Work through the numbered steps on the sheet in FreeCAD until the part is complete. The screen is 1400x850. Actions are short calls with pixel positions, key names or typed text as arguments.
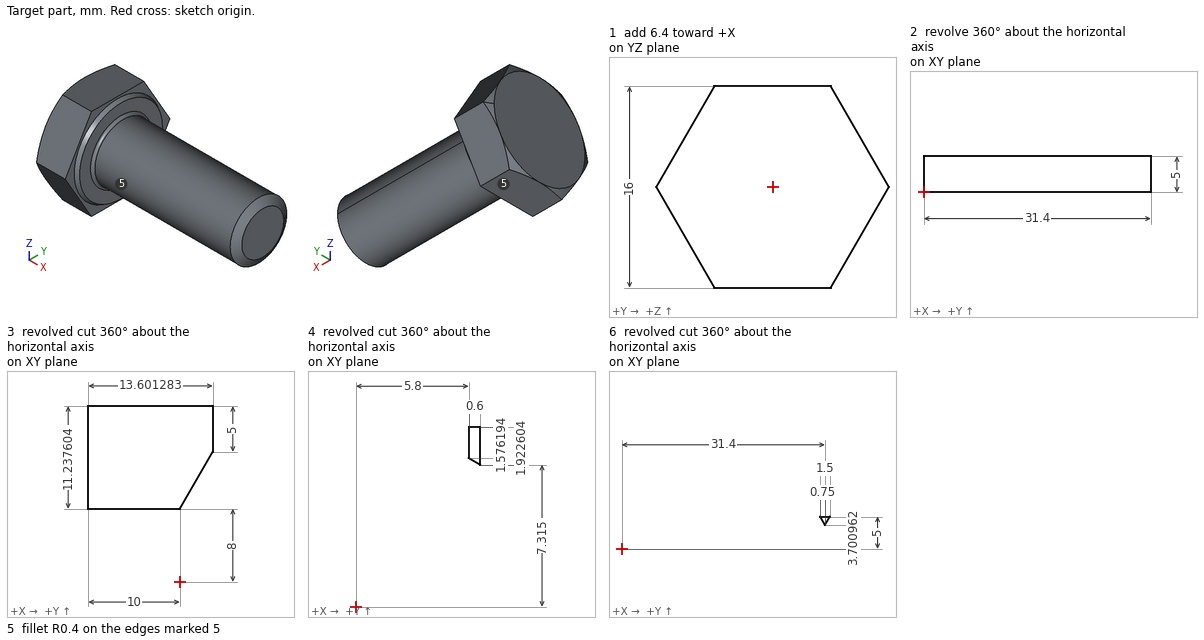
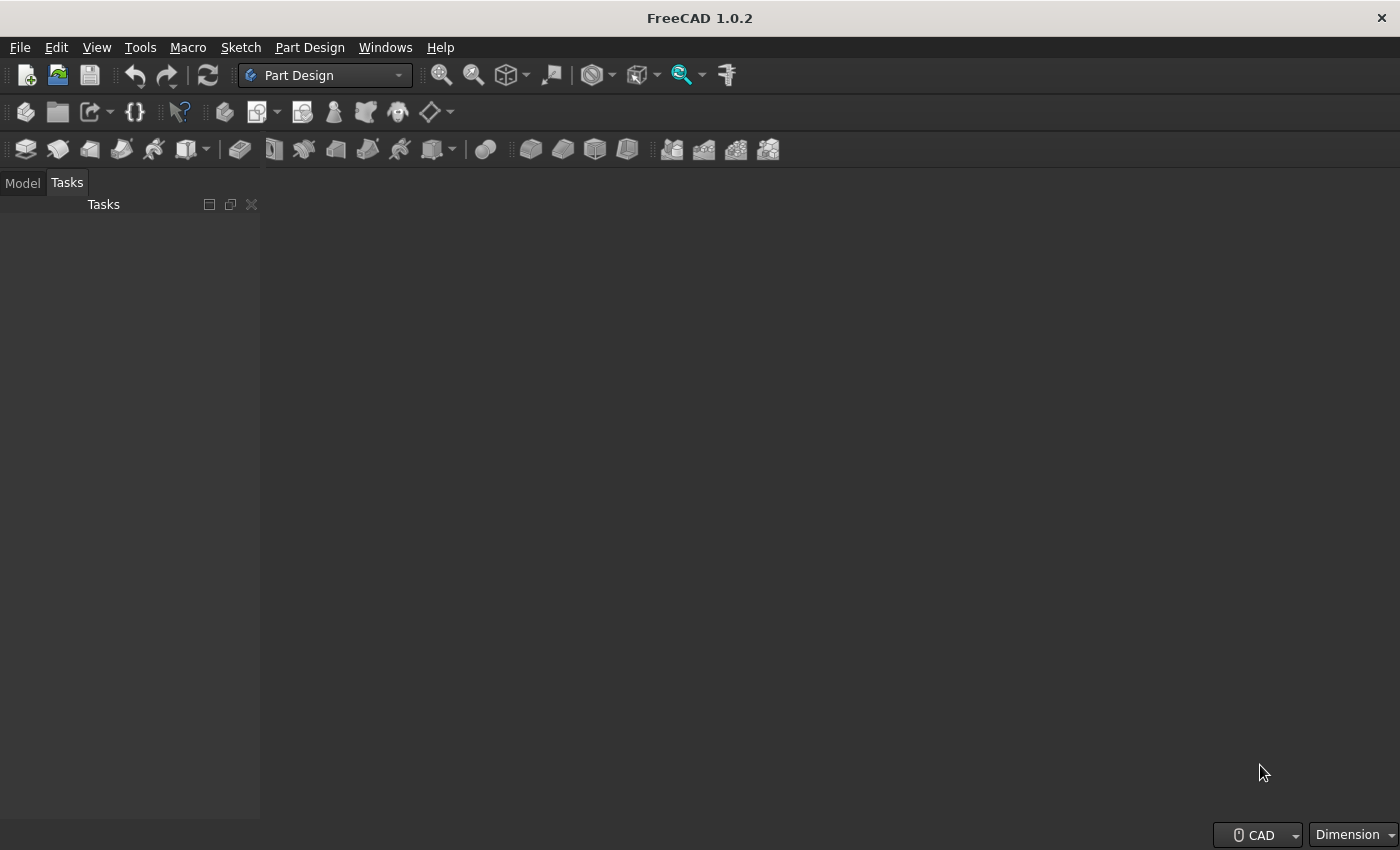
click(26, 76)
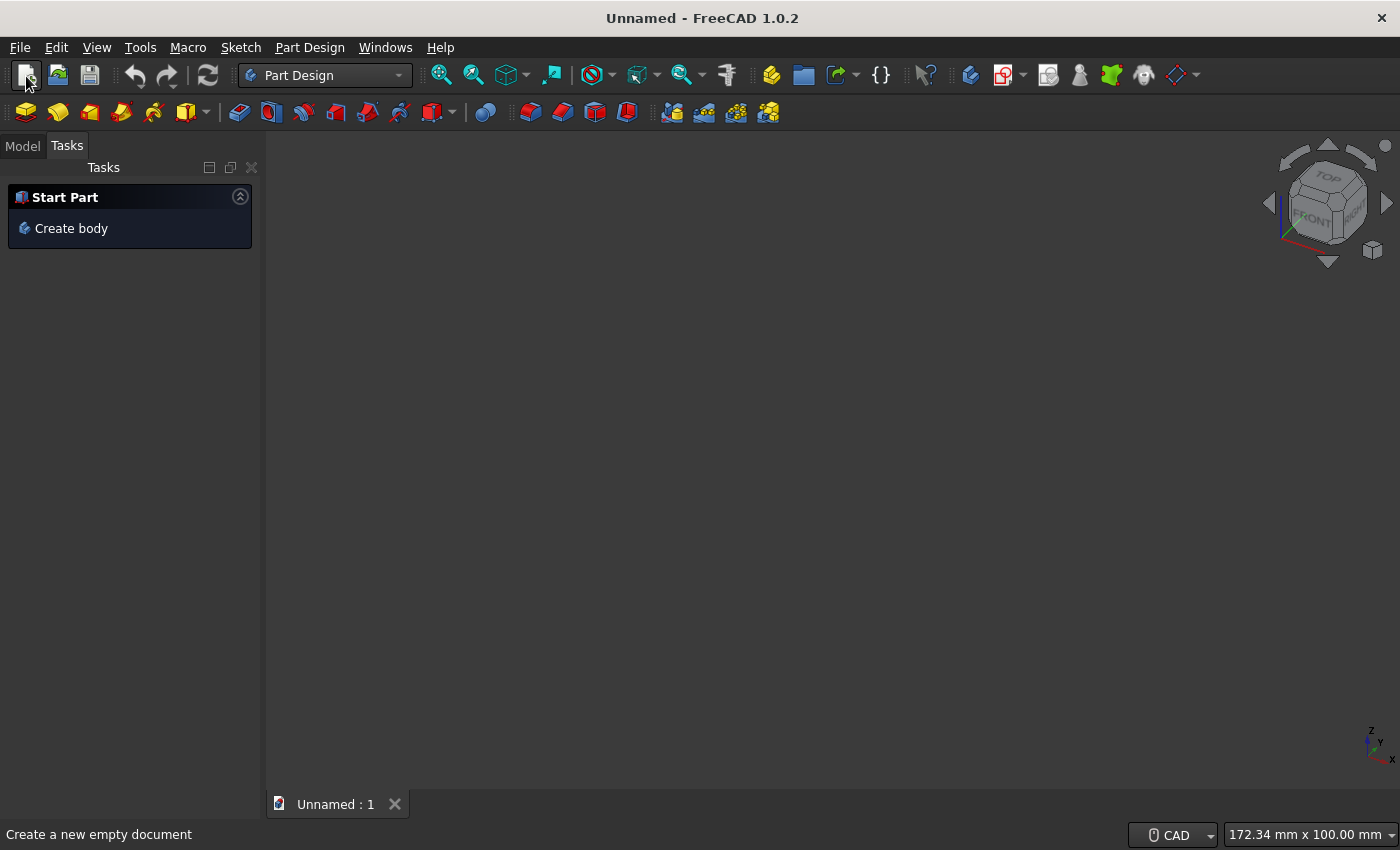
click(1004, 76)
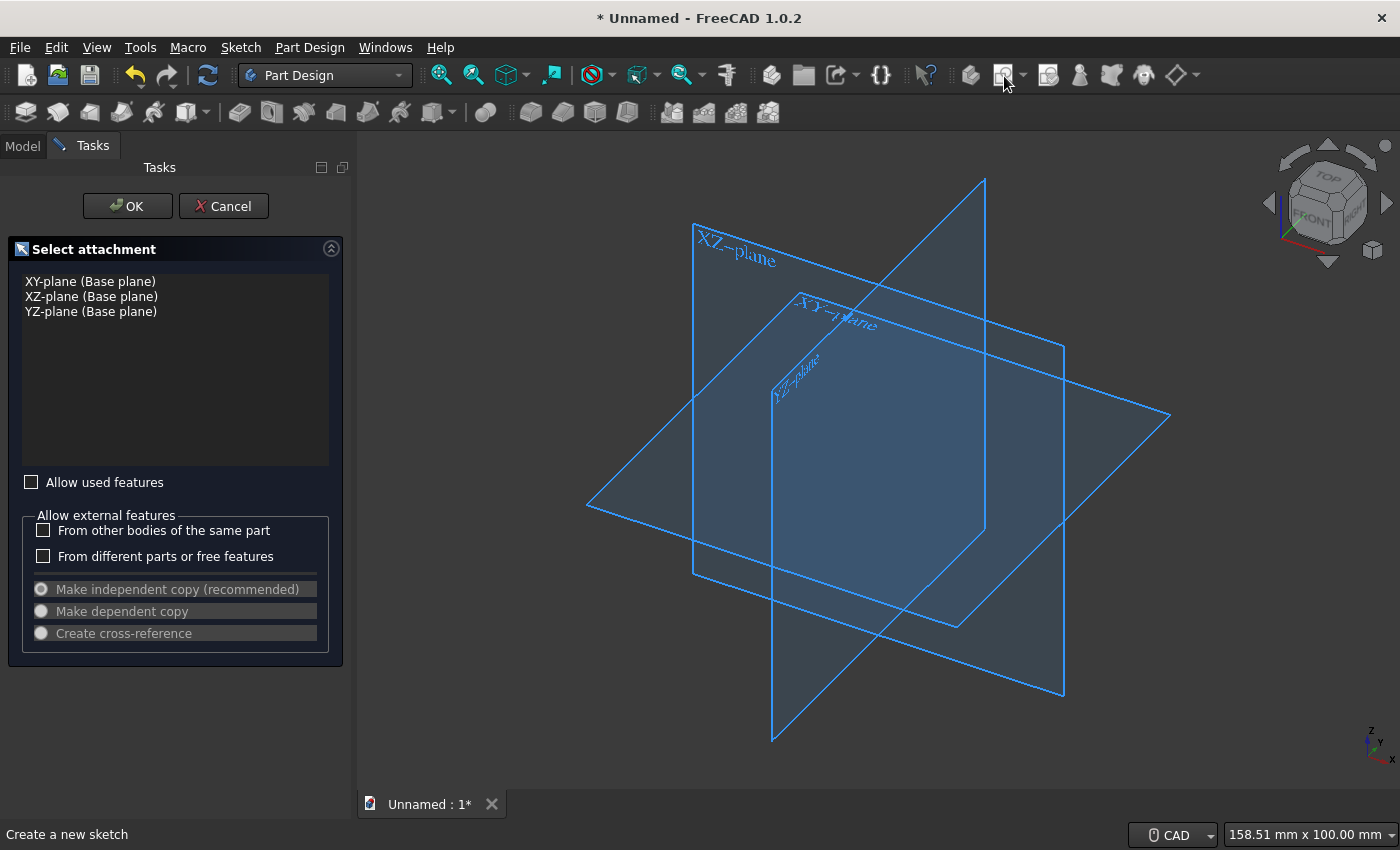
click(82, 312)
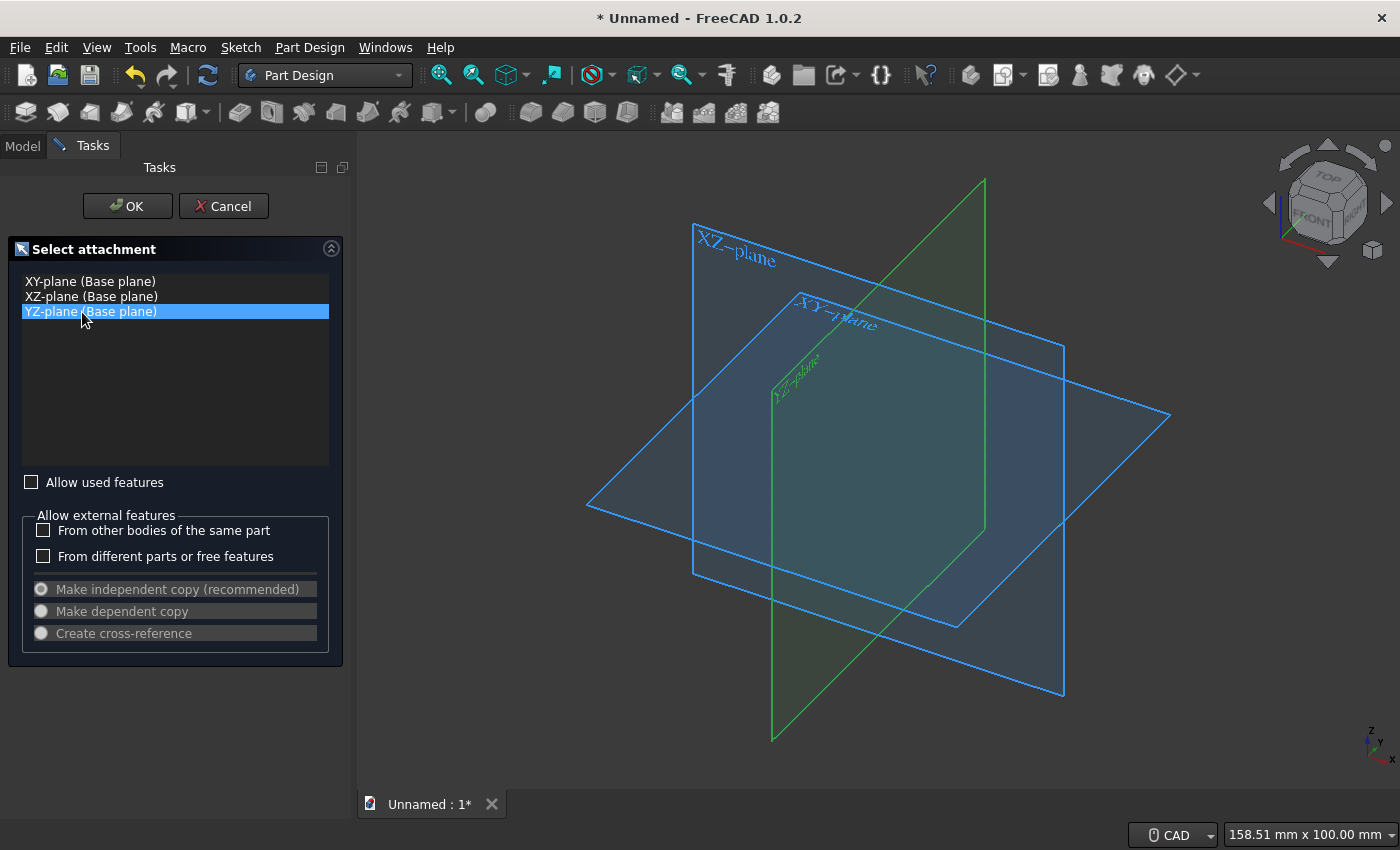
click(128, 206)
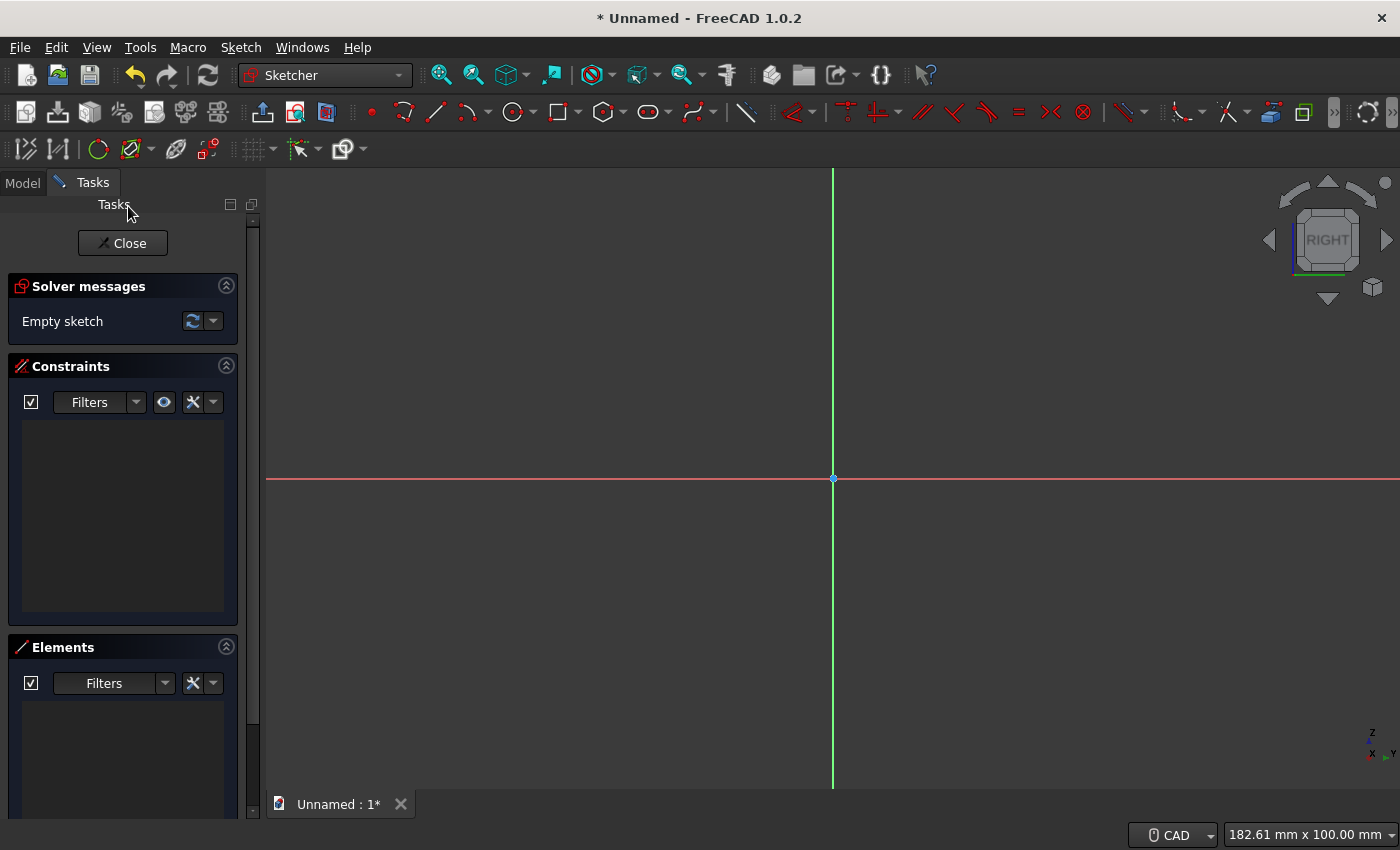
scroll(855, 479, up, 7)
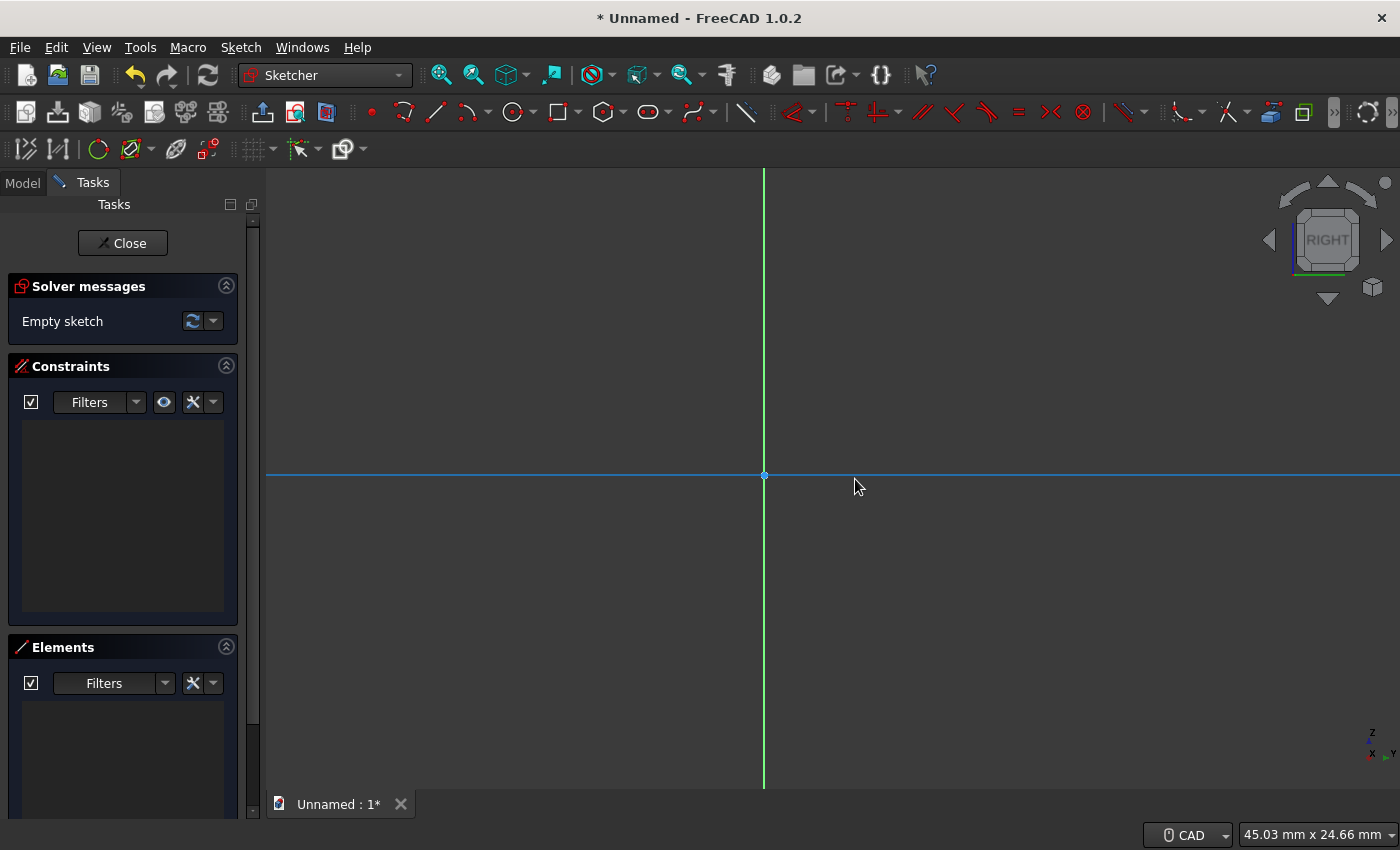
click(604, 112)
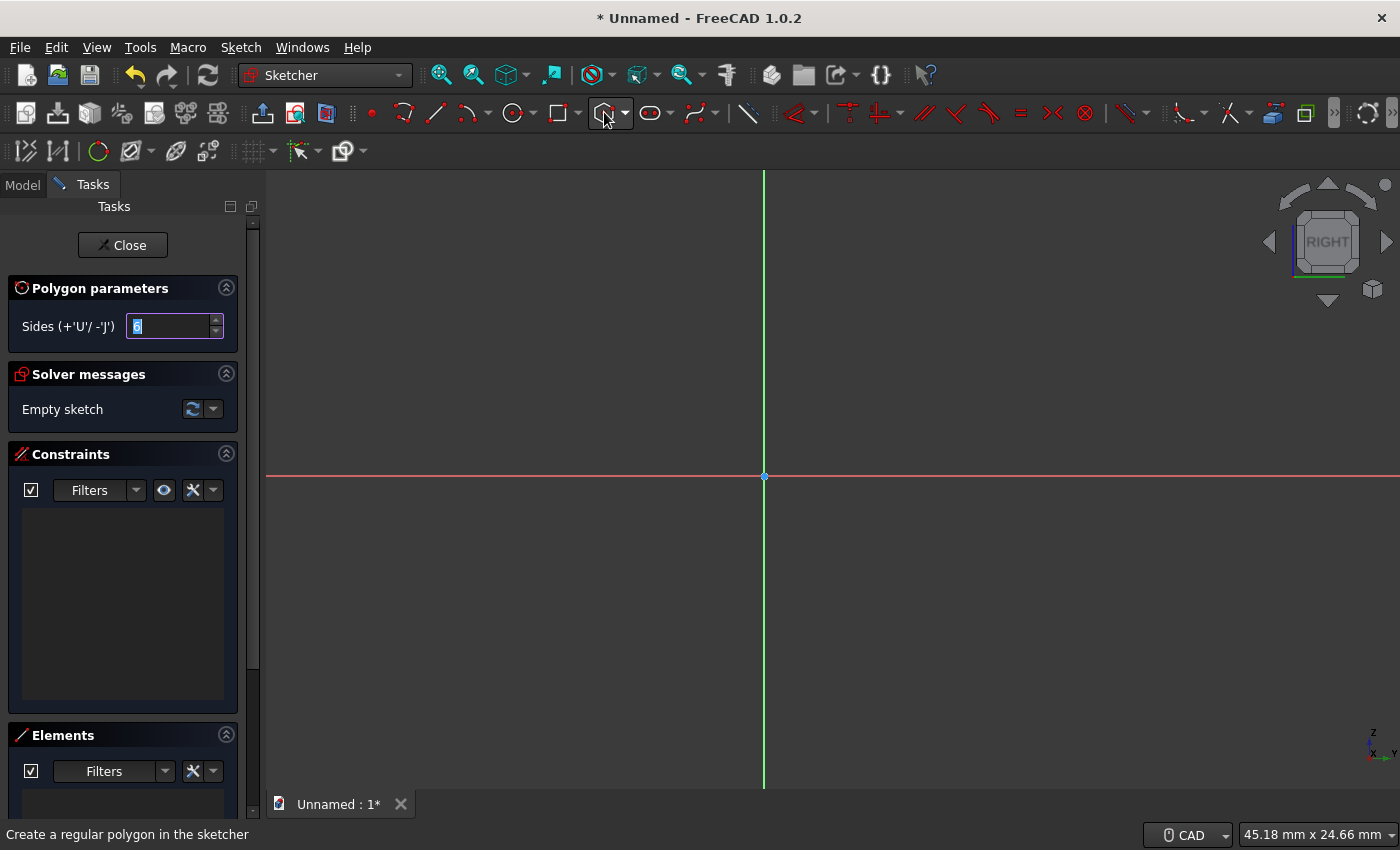
click(764, 476)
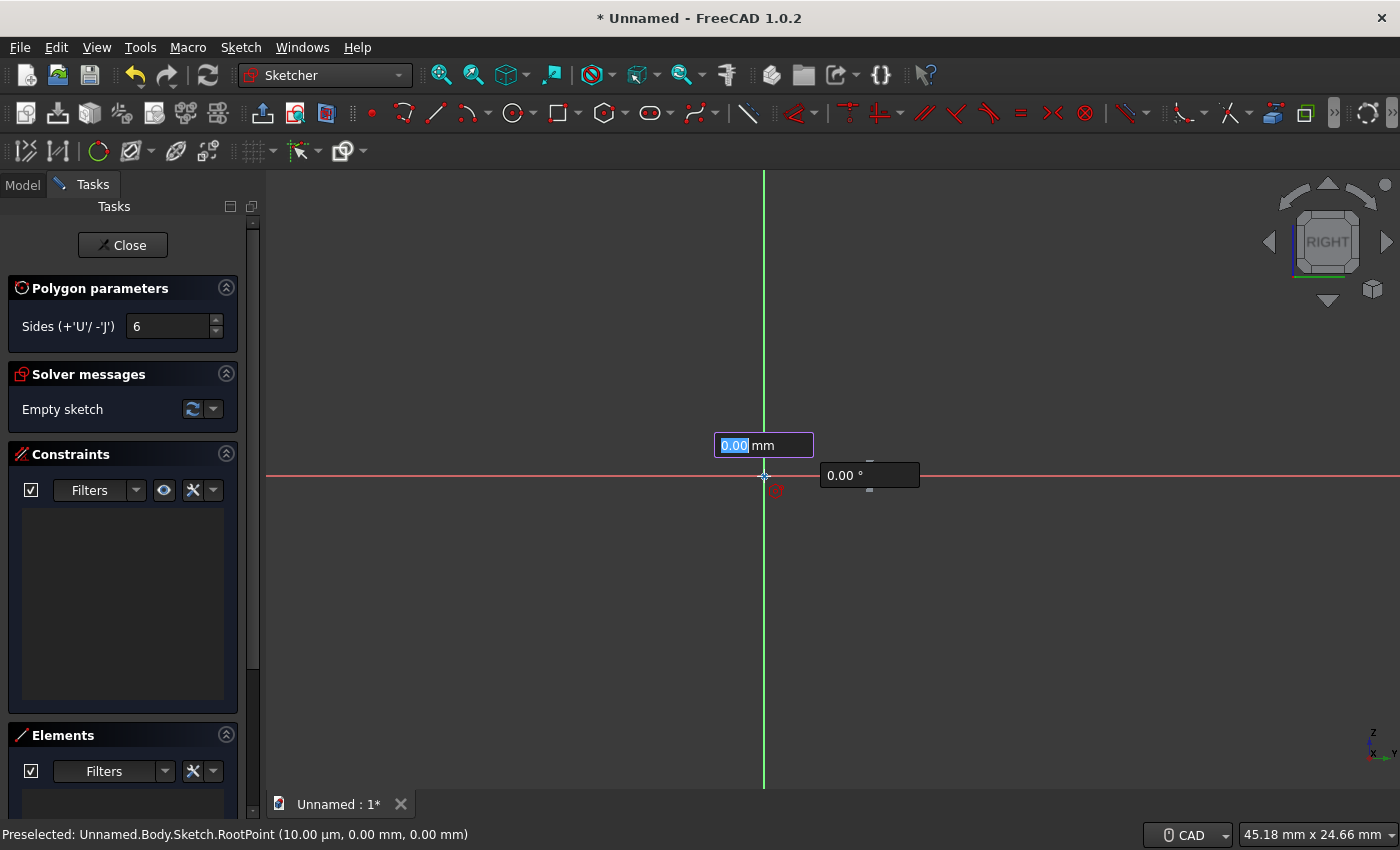
click(996, 476)
key(Escape)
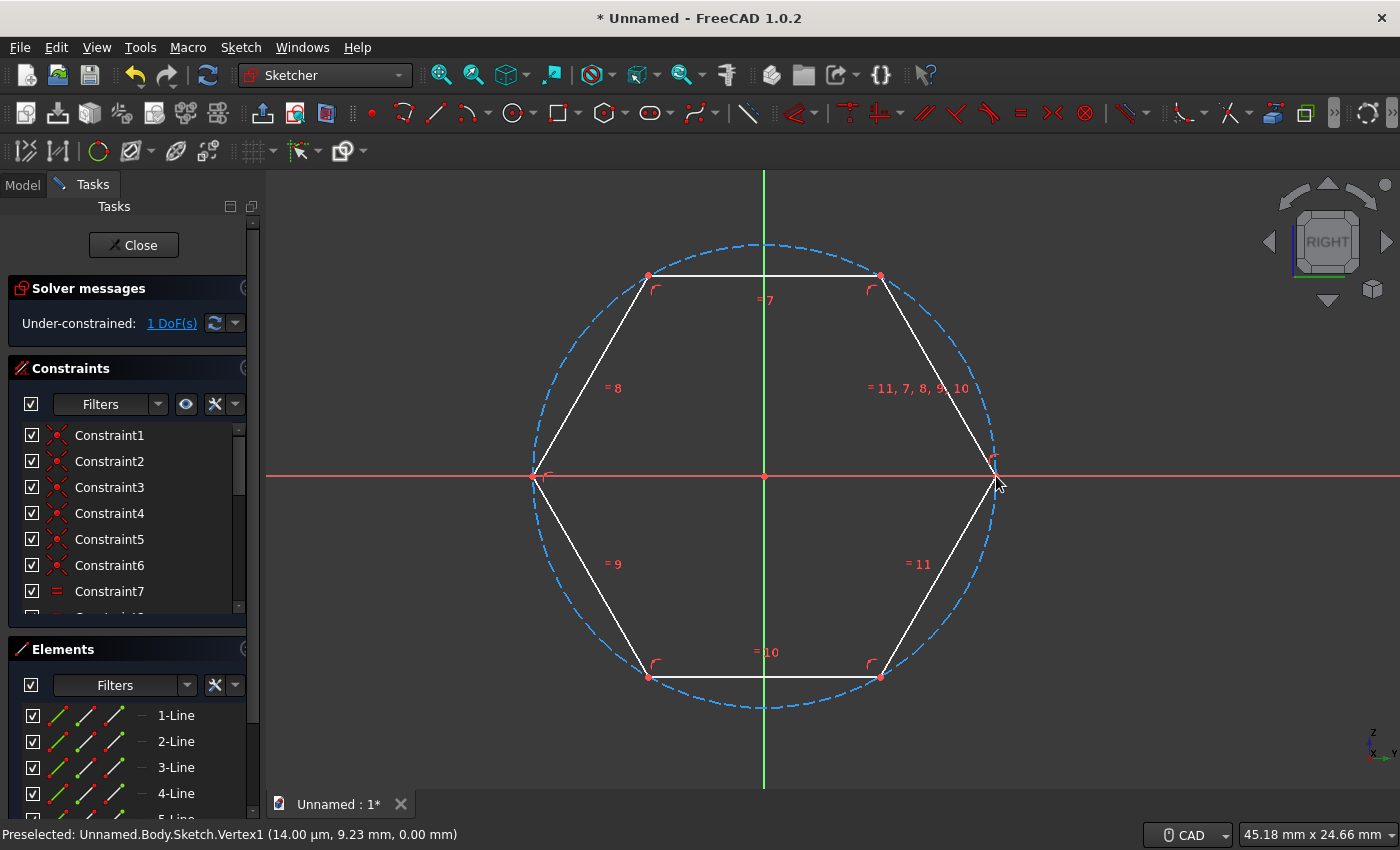
click(794, 114)